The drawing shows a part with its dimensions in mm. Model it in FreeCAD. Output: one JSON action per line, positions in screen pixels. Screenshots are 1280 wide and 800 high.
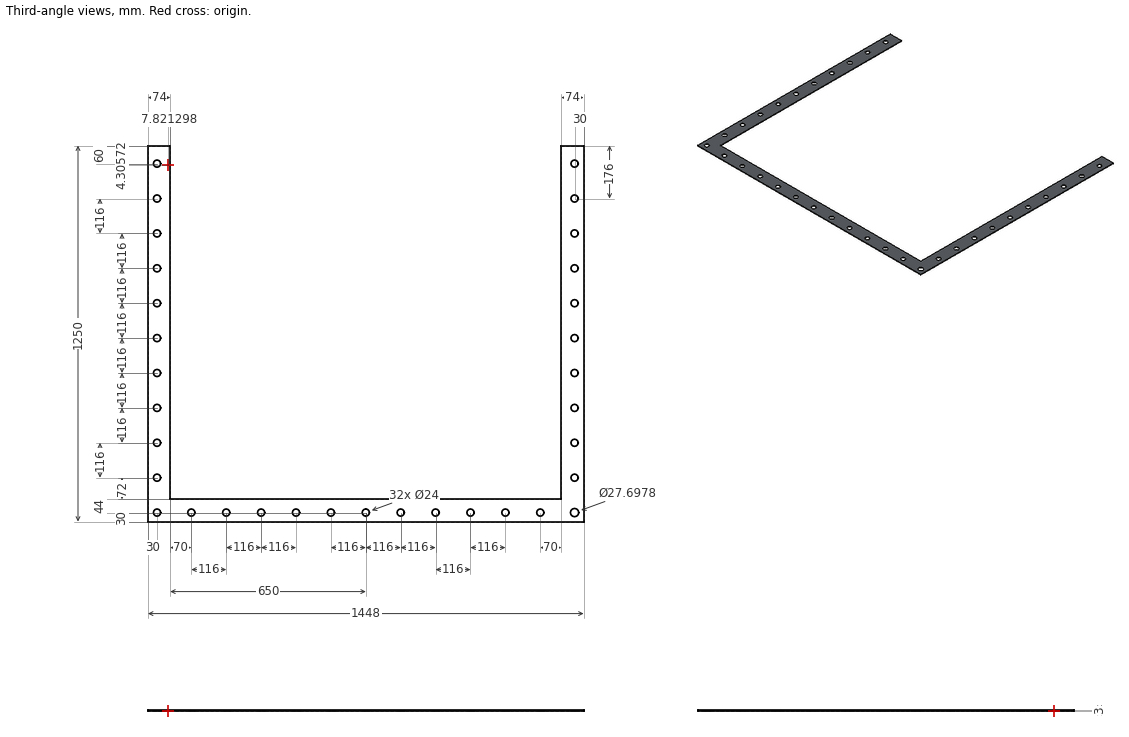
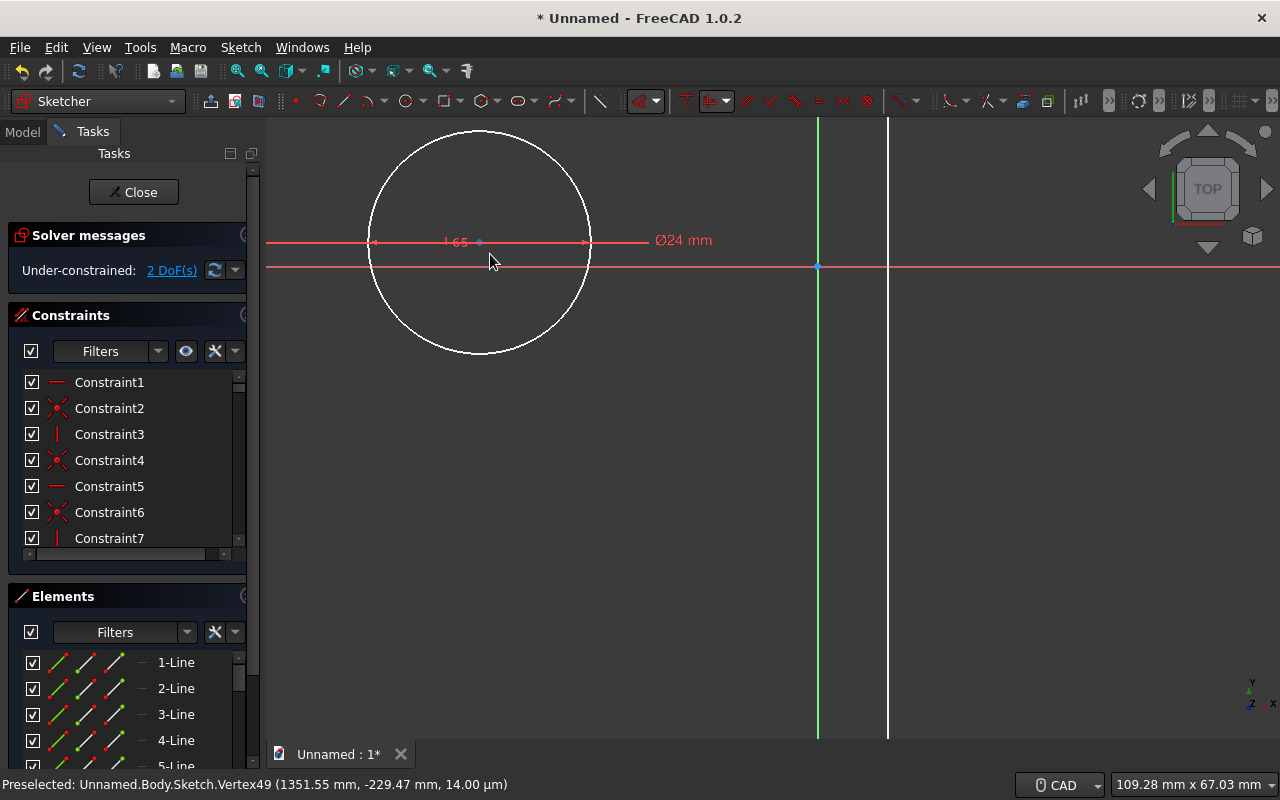
{"action": "left_click", "coordinate": [480, 243]}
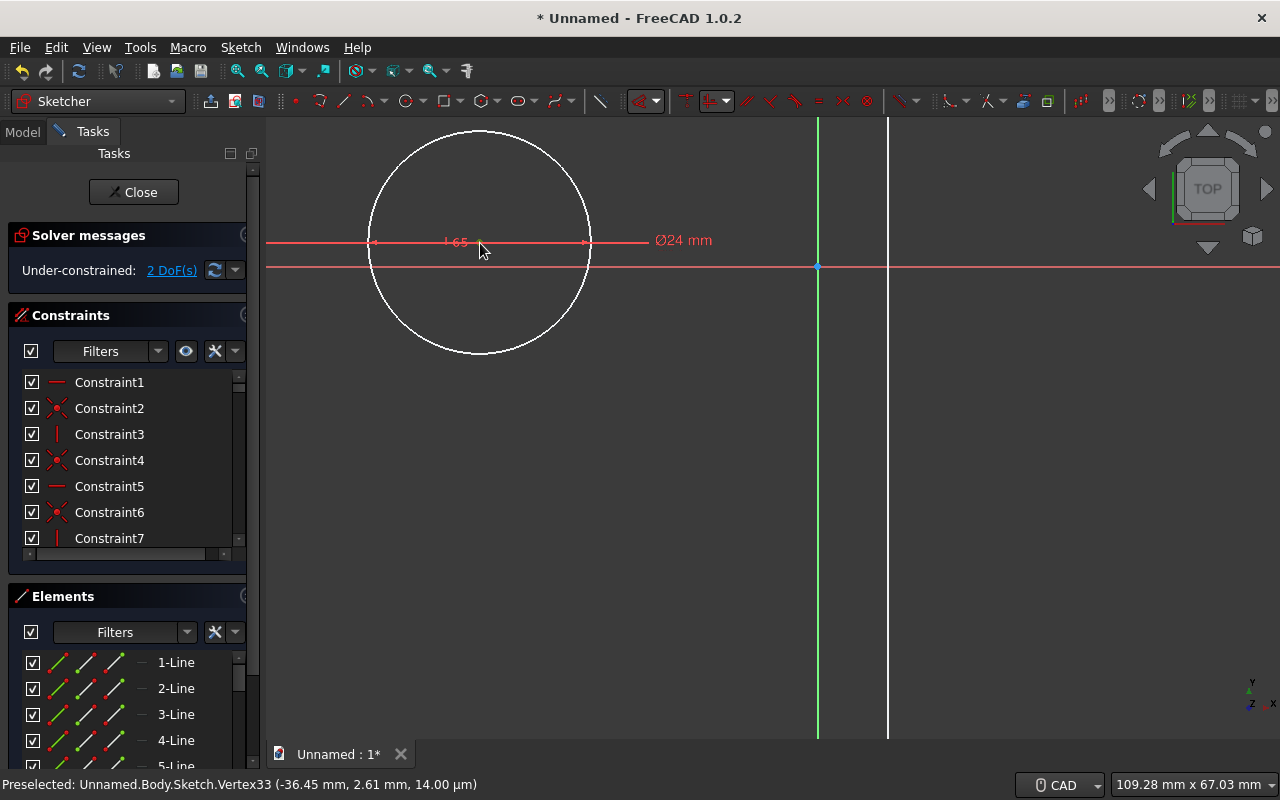
{"action": "left_click", "coordinate": [658, 102]}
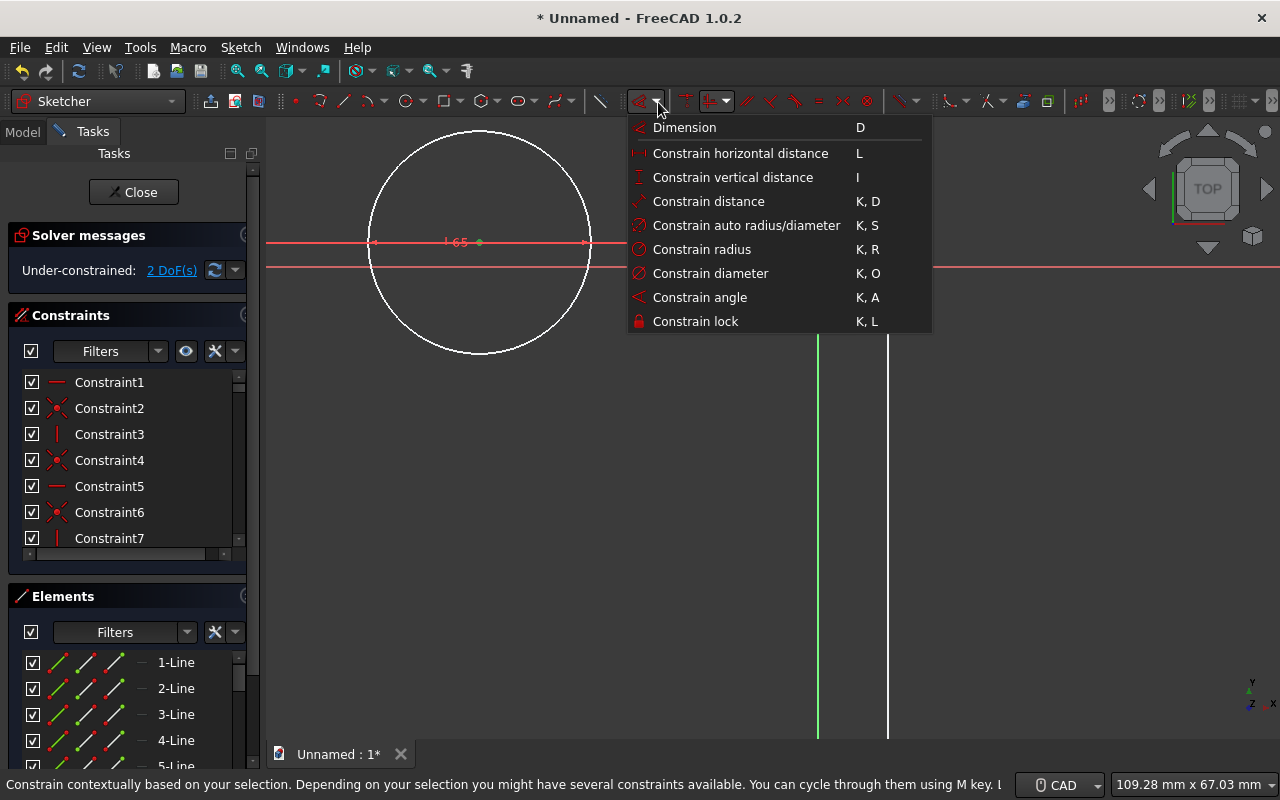
{"action": "left_click", "coordinate": [780, 177]}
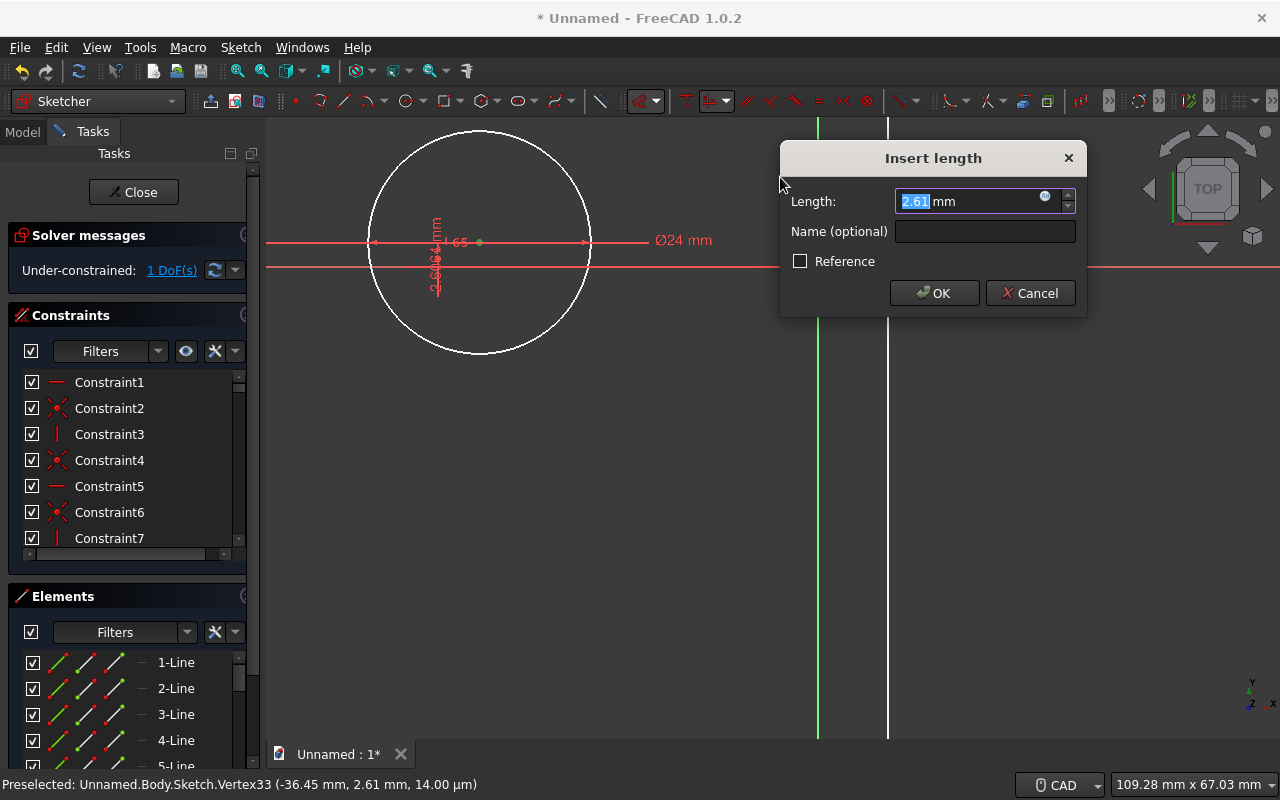
{"action": "type", "text": "4.30572"}
{"action": "key", "text": "Return"}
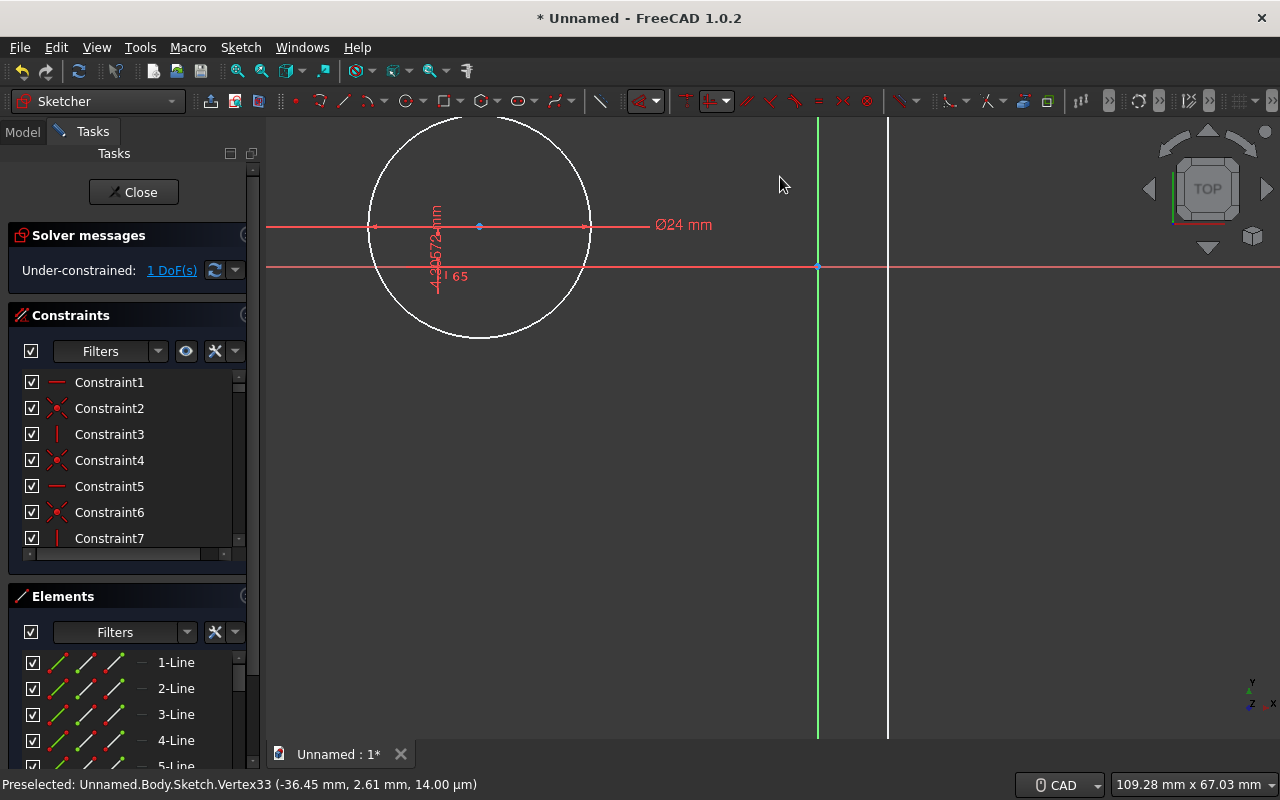
{"action": "scroll", "coordinate": [440, 214], "scroll_direction": "down", "scroll_amount": 16}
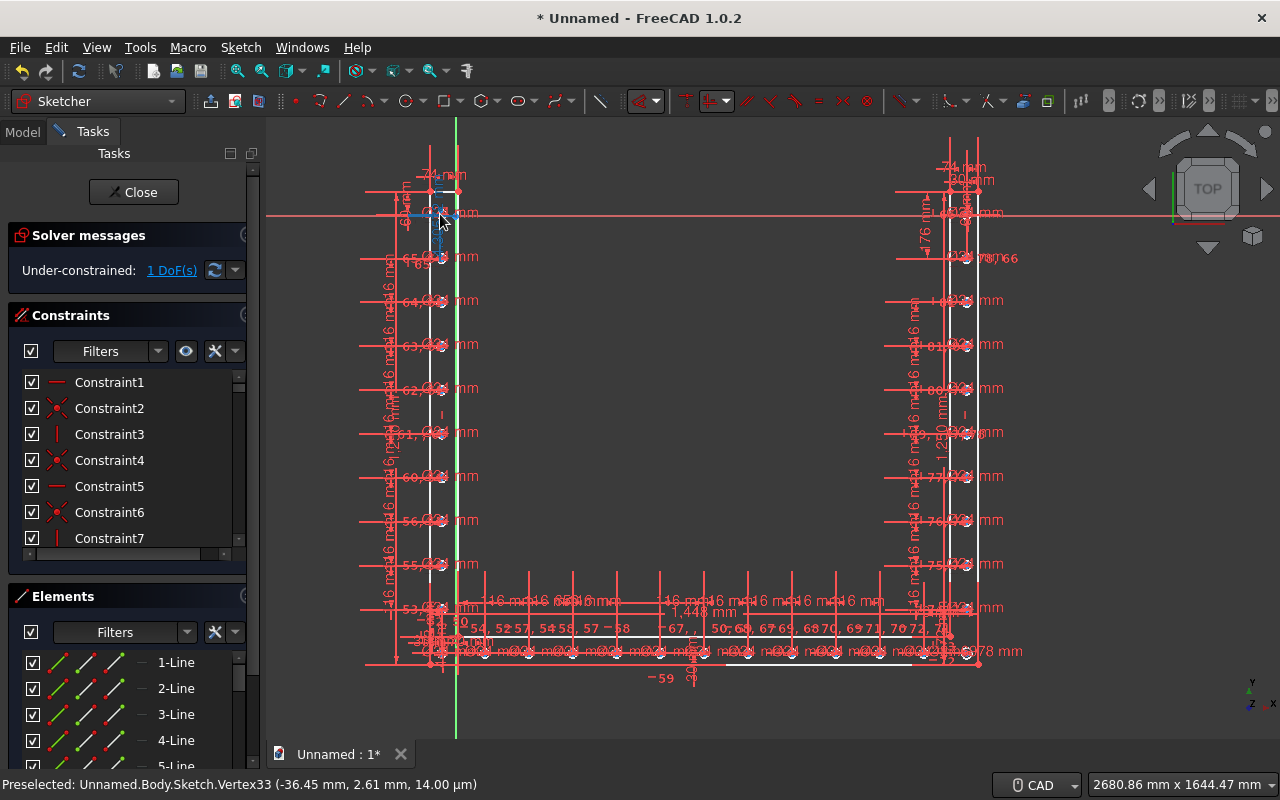
{"action": "scroll", "coordinate": [458, 192], "scroll_direction": "up", "scroll_amount": 13}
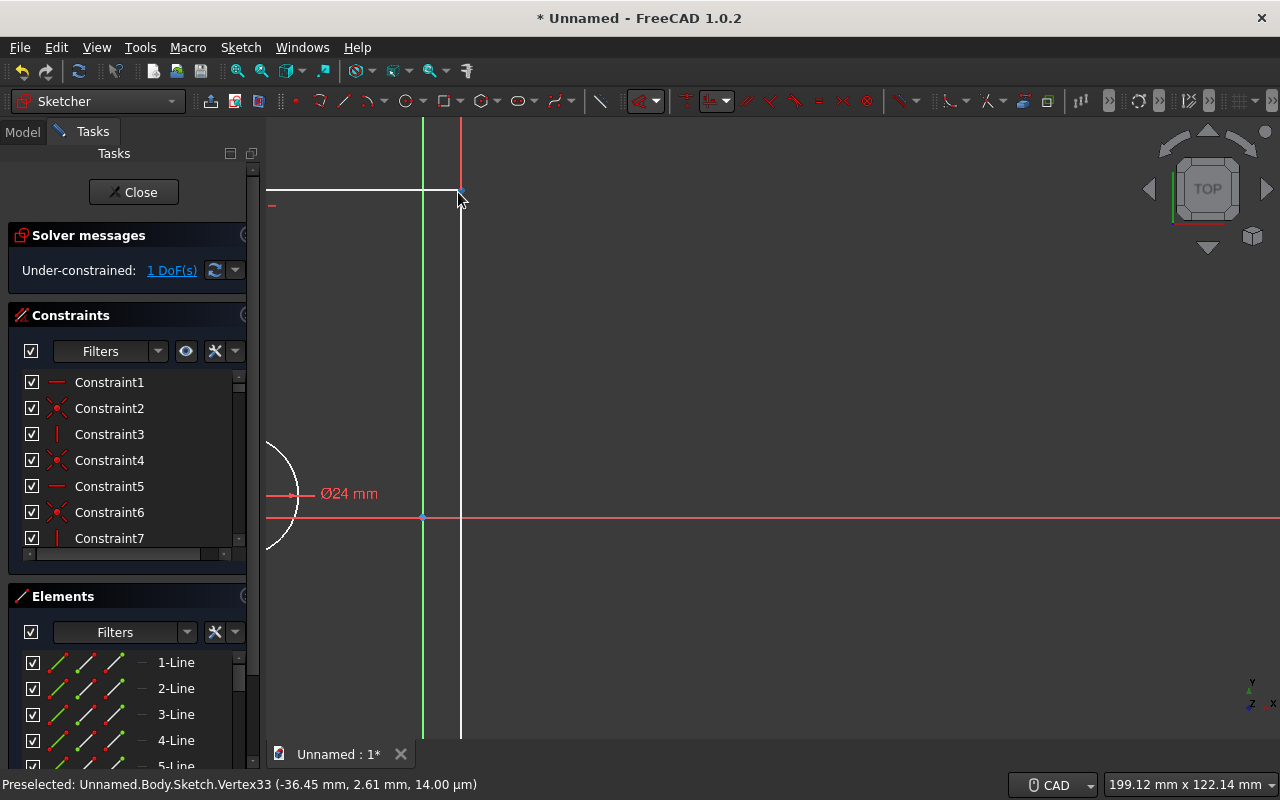
{"action": "left_click", "coordinate": [461, 190]}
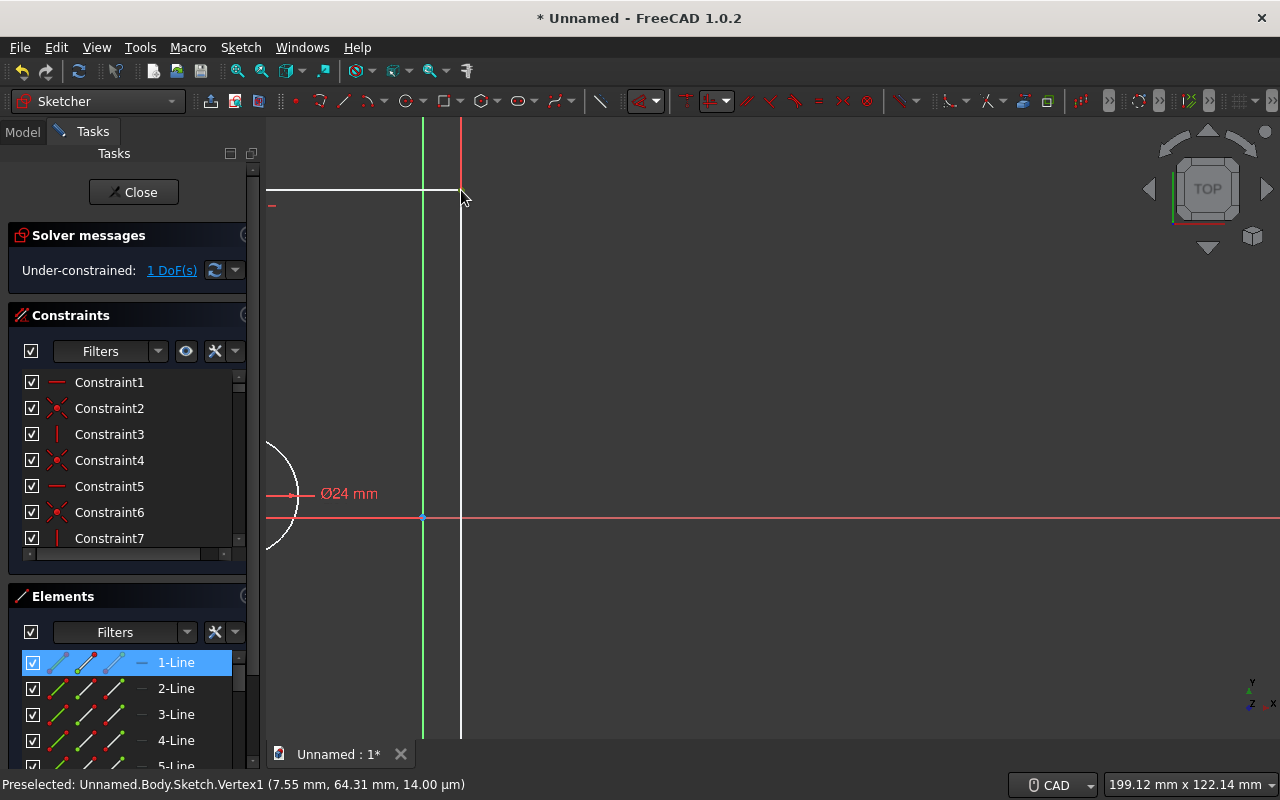
{"action": "left_click", "coordinate": [658, 102]}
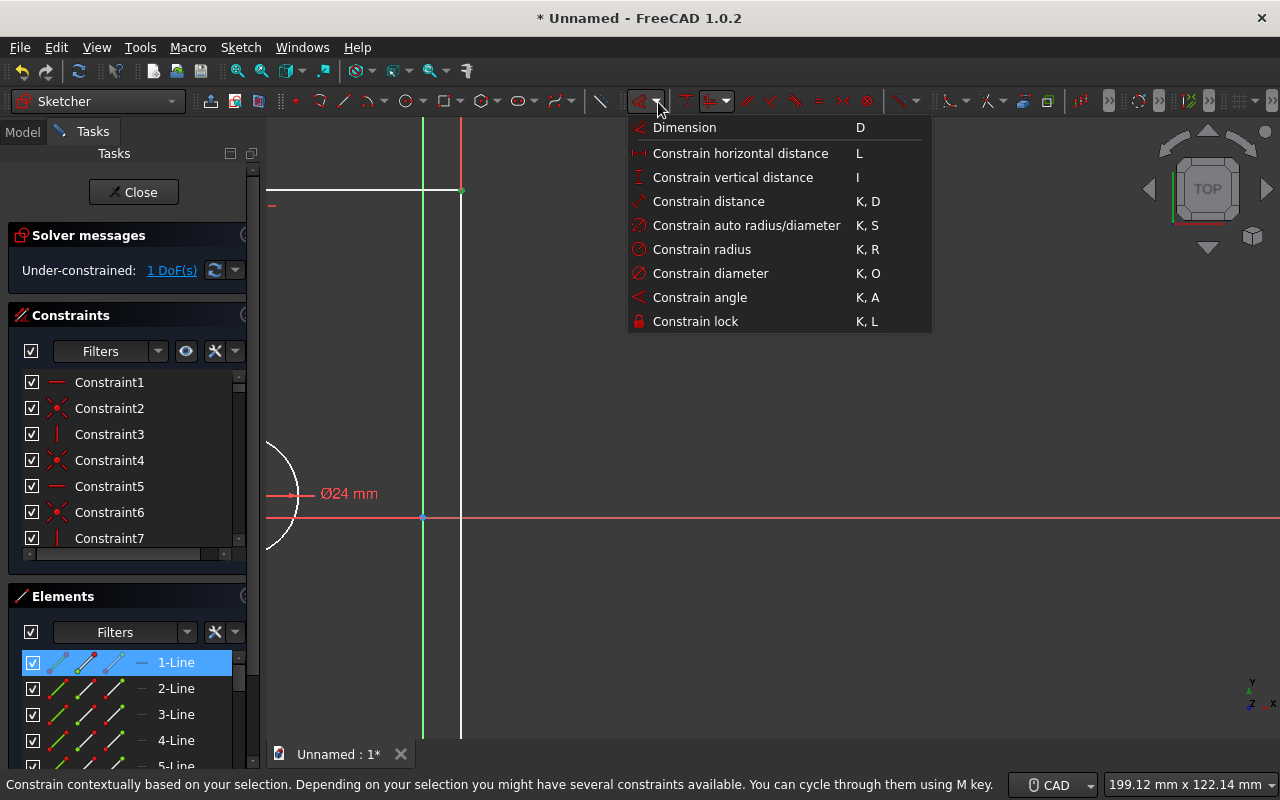
{"action": "left_click", "coordinate": [780, 153]}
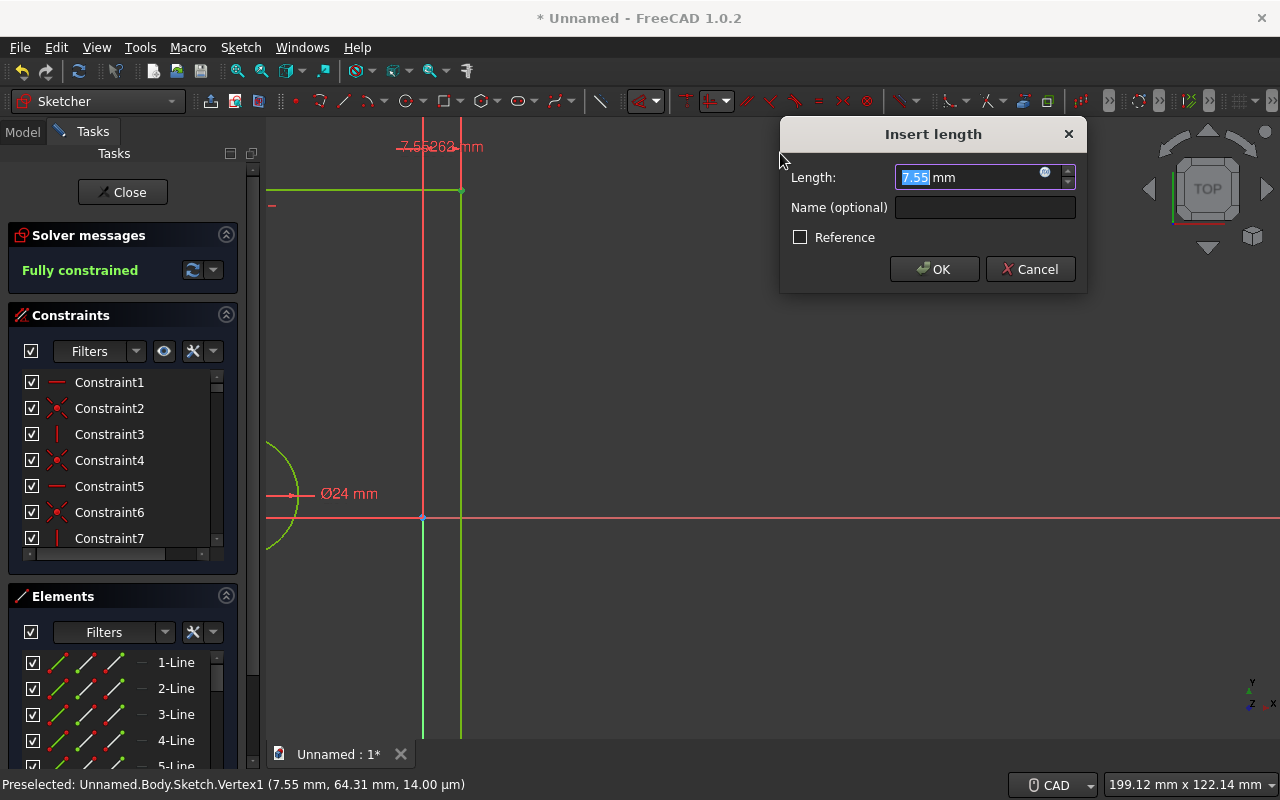
{"action": "type", "text": "7.821298"}
{"action": "key", "text": "Return"}